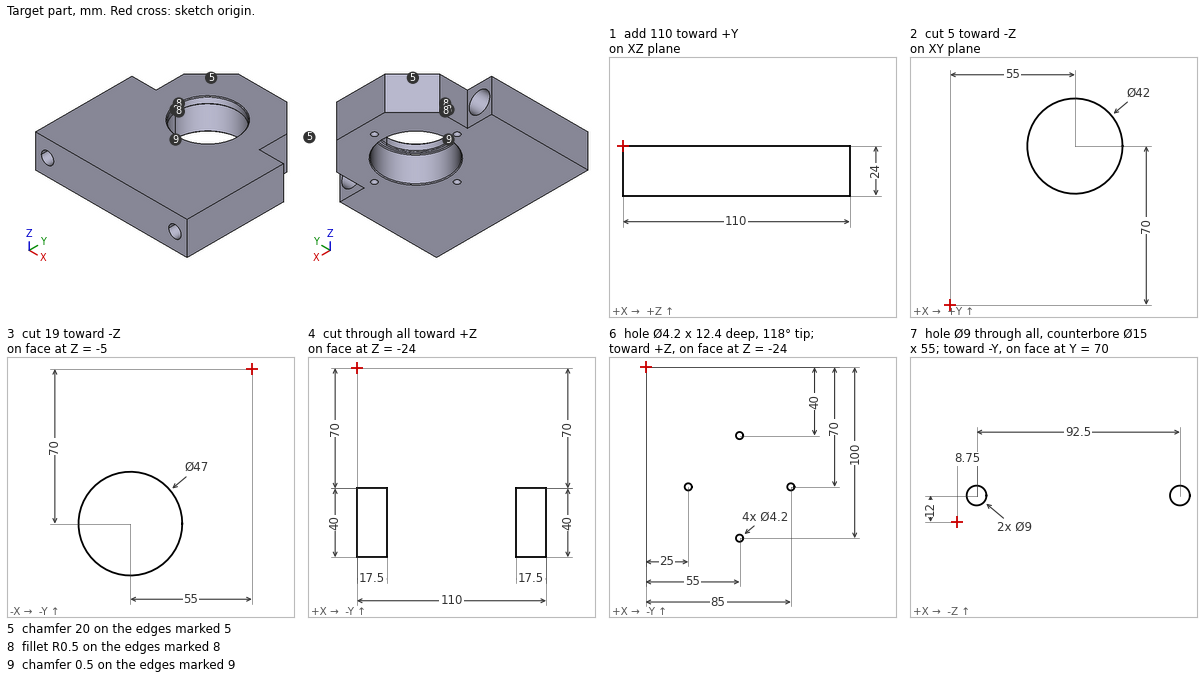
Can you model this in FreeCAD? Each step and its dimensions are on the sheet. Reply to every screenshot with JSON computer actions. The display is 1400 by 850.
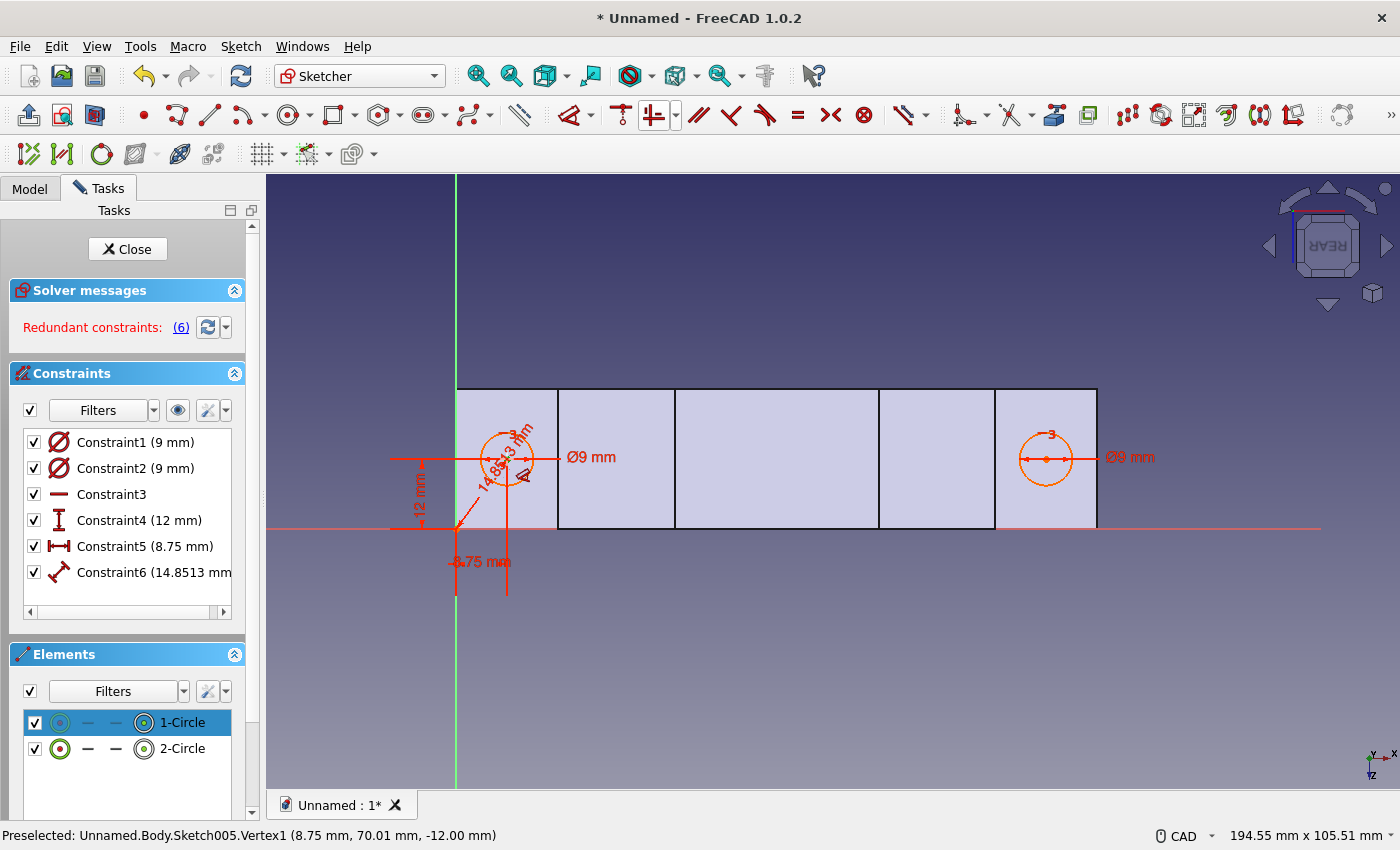
{"action": "left_click", "coordinate": [1046, 459]}
{"action": "left_click", "coordinate": [777, 425]}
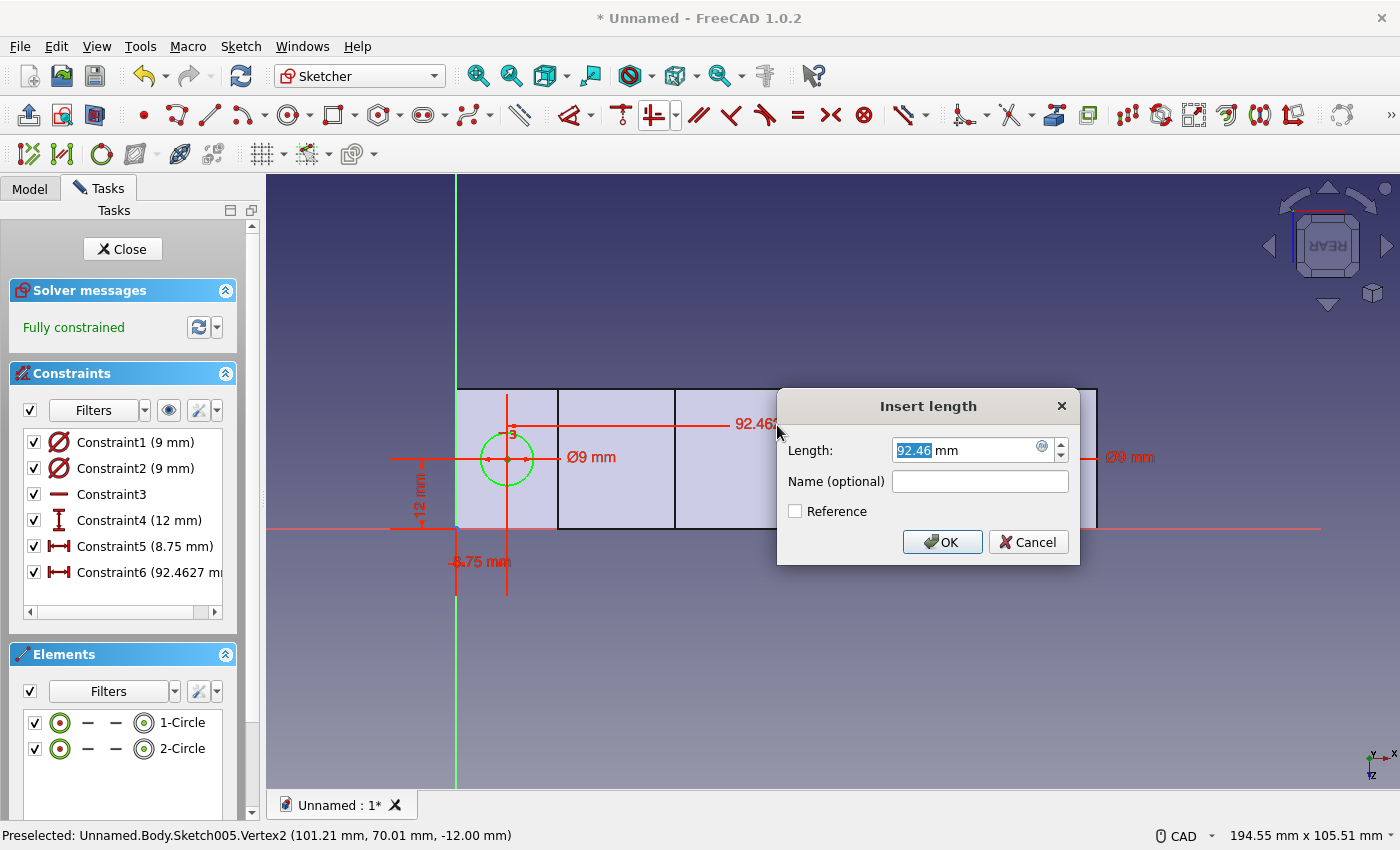
{"action": "type", "text": "92.5"}
{"action": "key", "text": "Return"}
{"action": "key", "text": "Escape"}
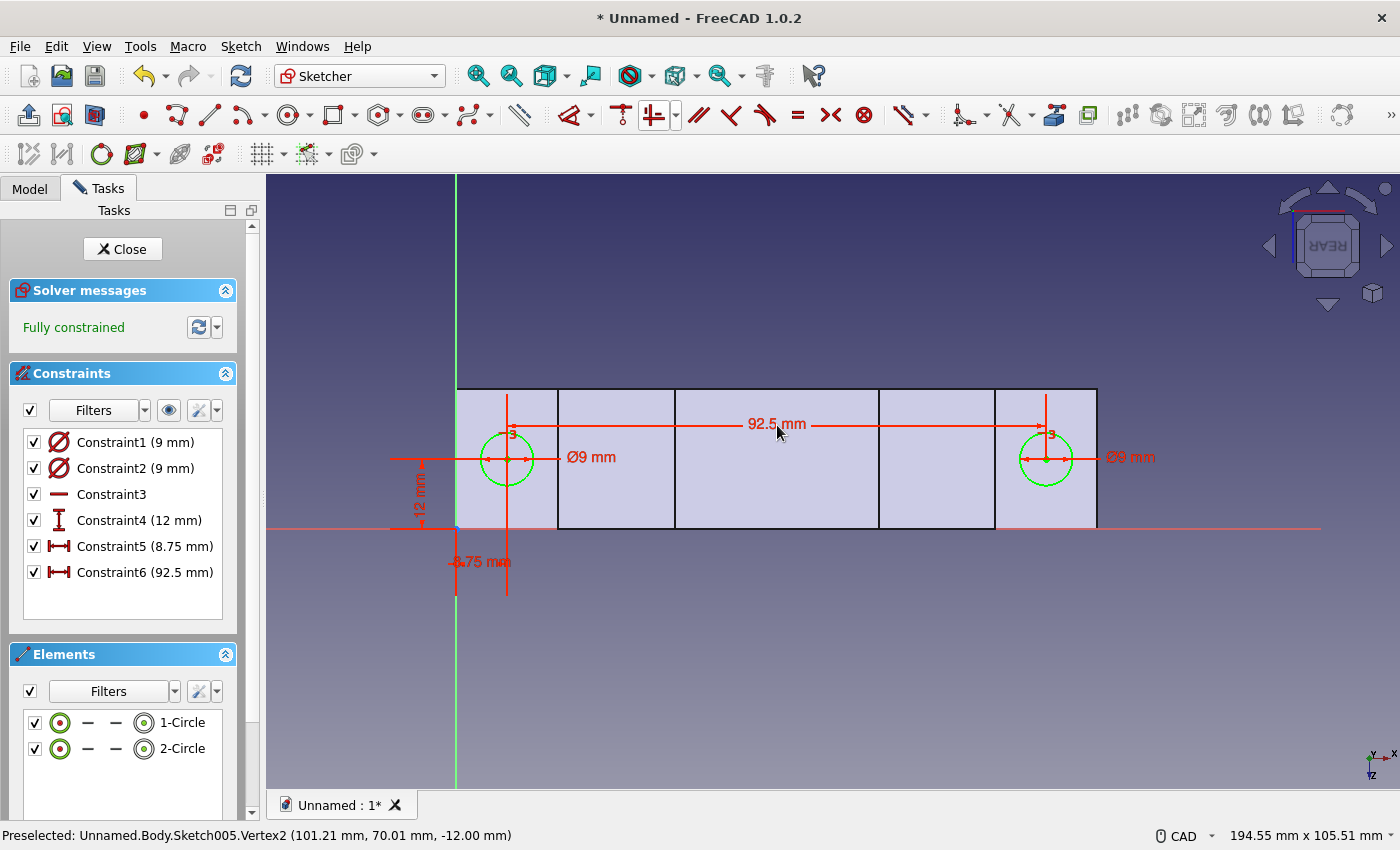
{"action": "left_click", "coordinate": [123, 249]}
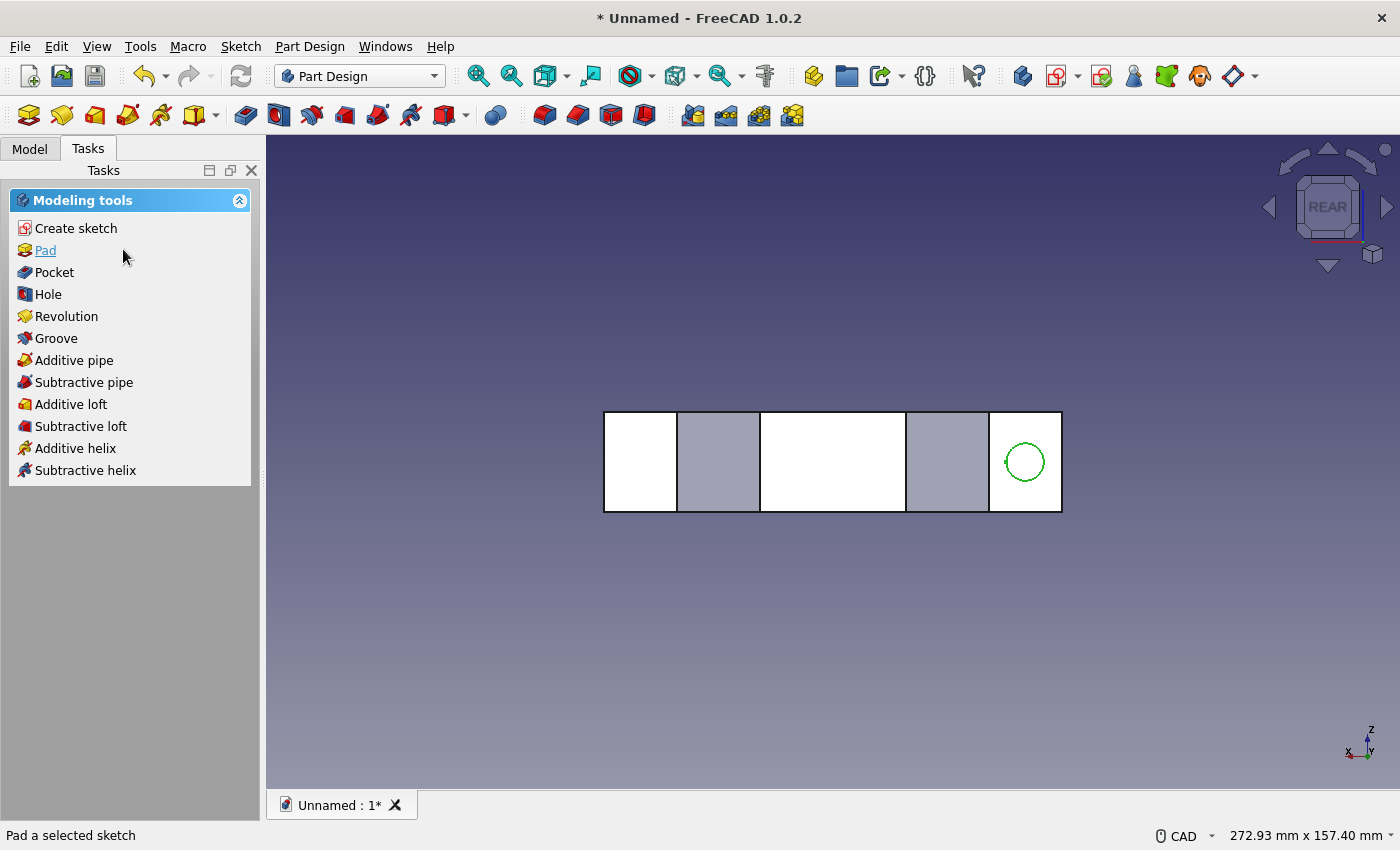
{"action": "left_click", "coordinate": [279, 116]}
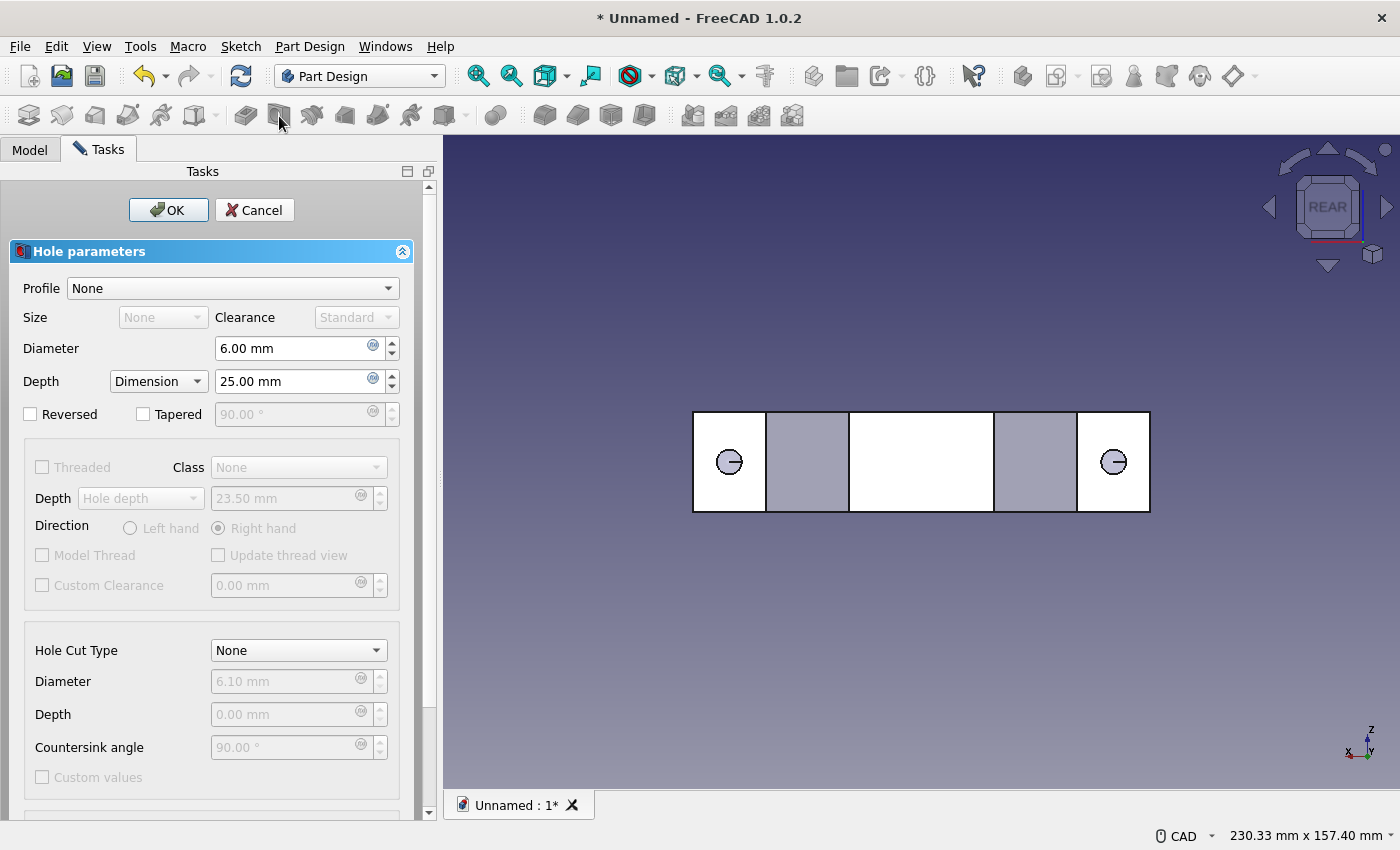
{"action": "triple_click", "coordinate": [300, 348]}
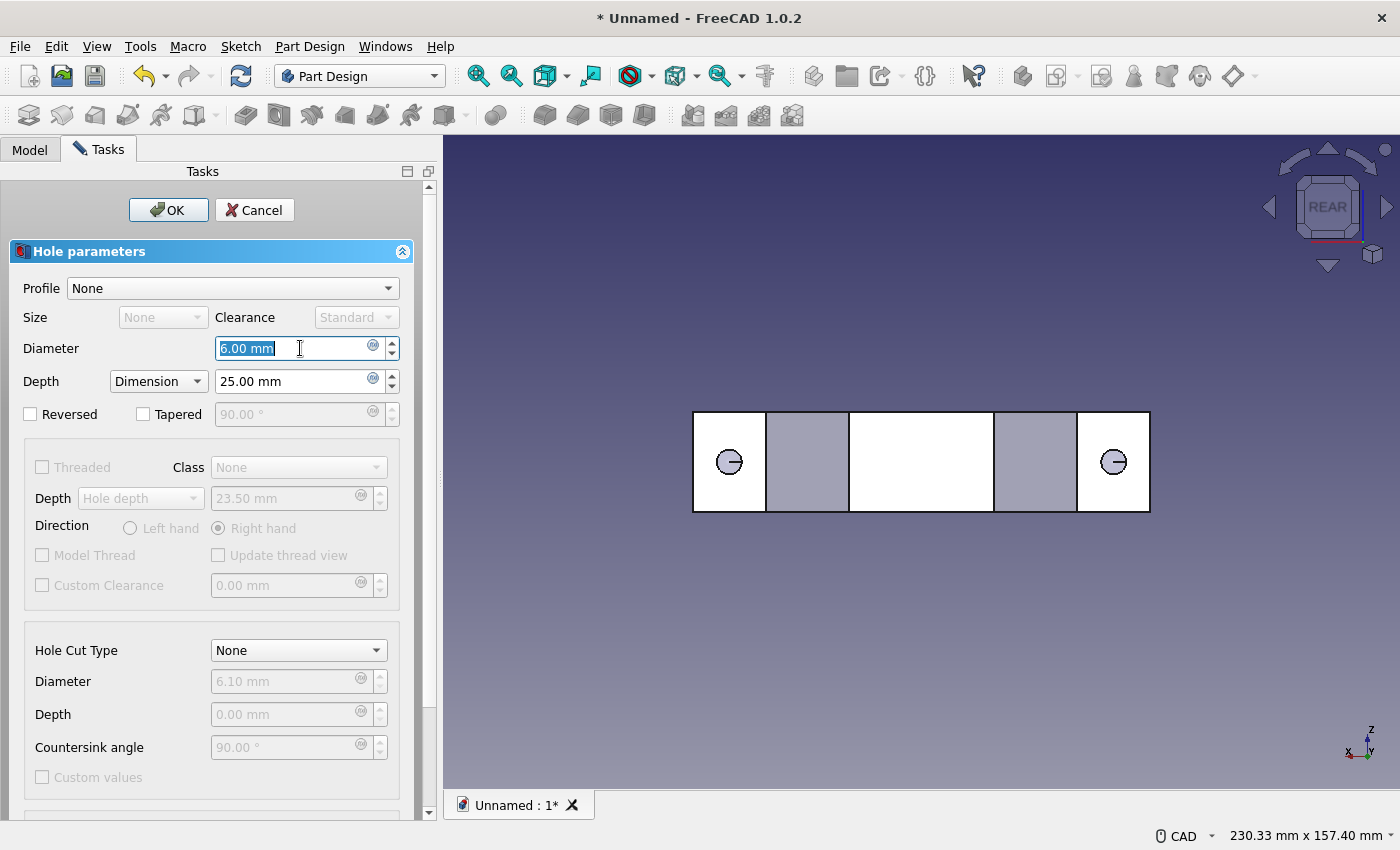
{"action": "type", "text": "9"}
{"action": "key", "text": "Tab"}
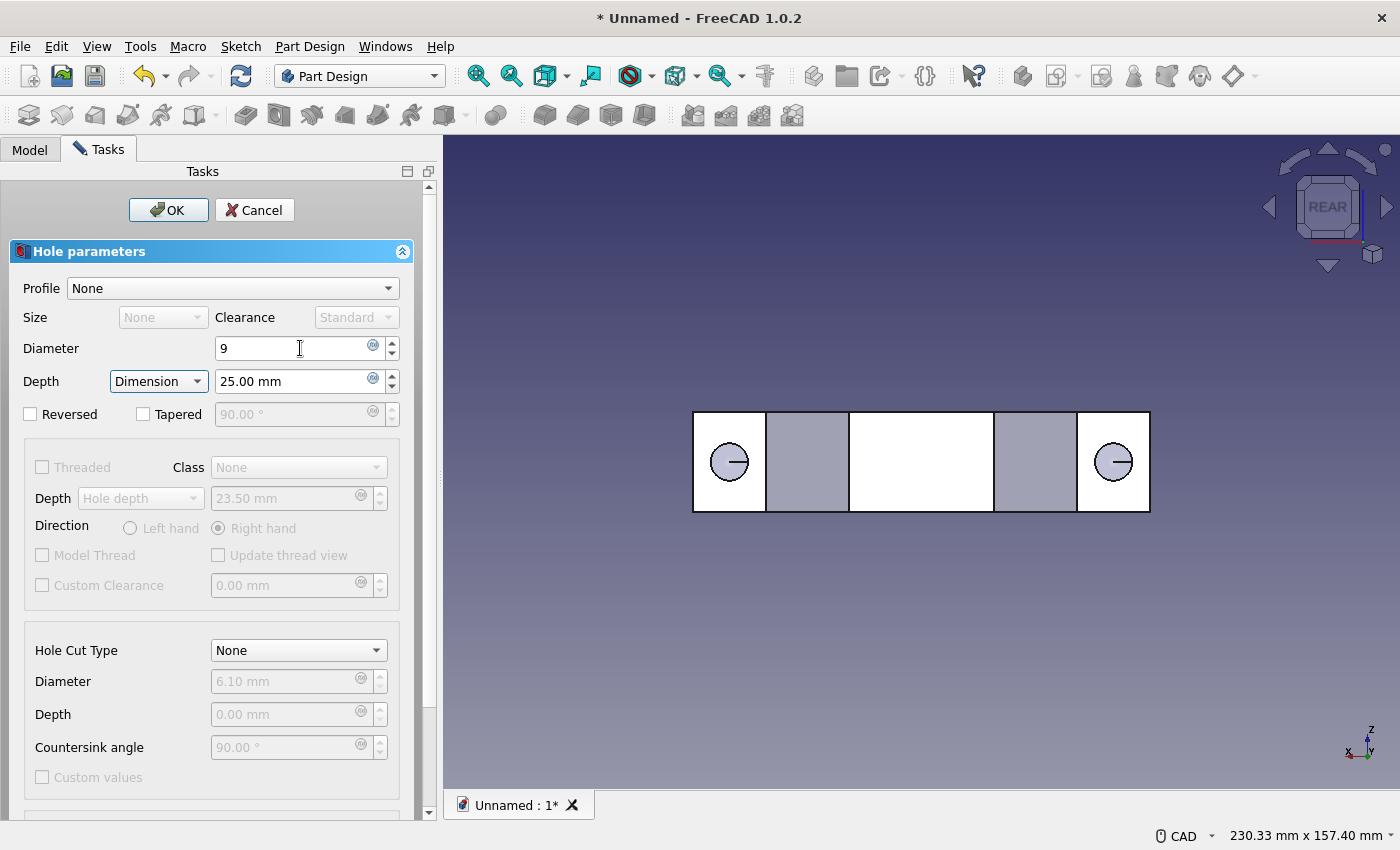
{"action": "left_click", "coordinate": [160, 382]}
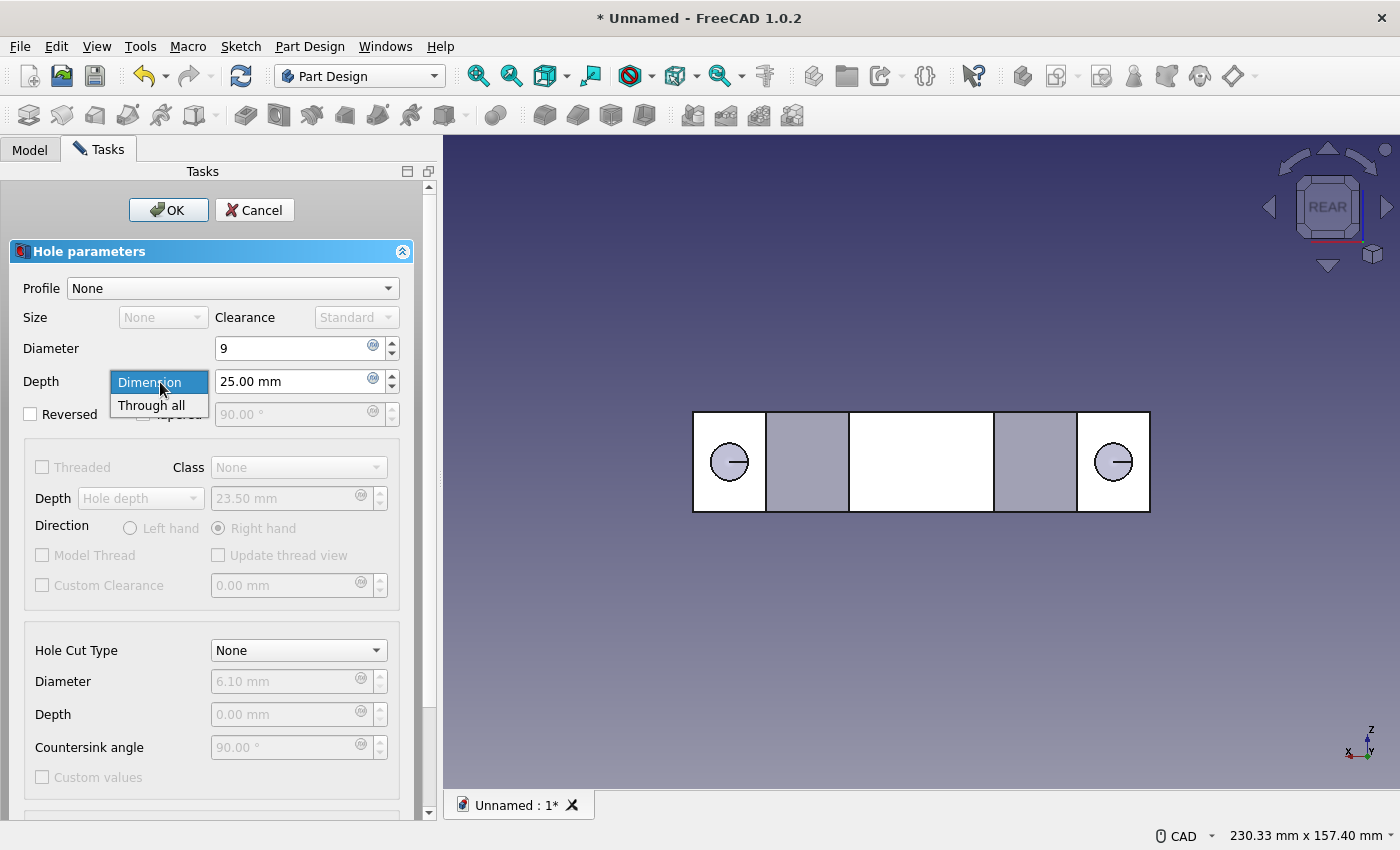
{"action": "left_click", "coordinate": [158, 406]}